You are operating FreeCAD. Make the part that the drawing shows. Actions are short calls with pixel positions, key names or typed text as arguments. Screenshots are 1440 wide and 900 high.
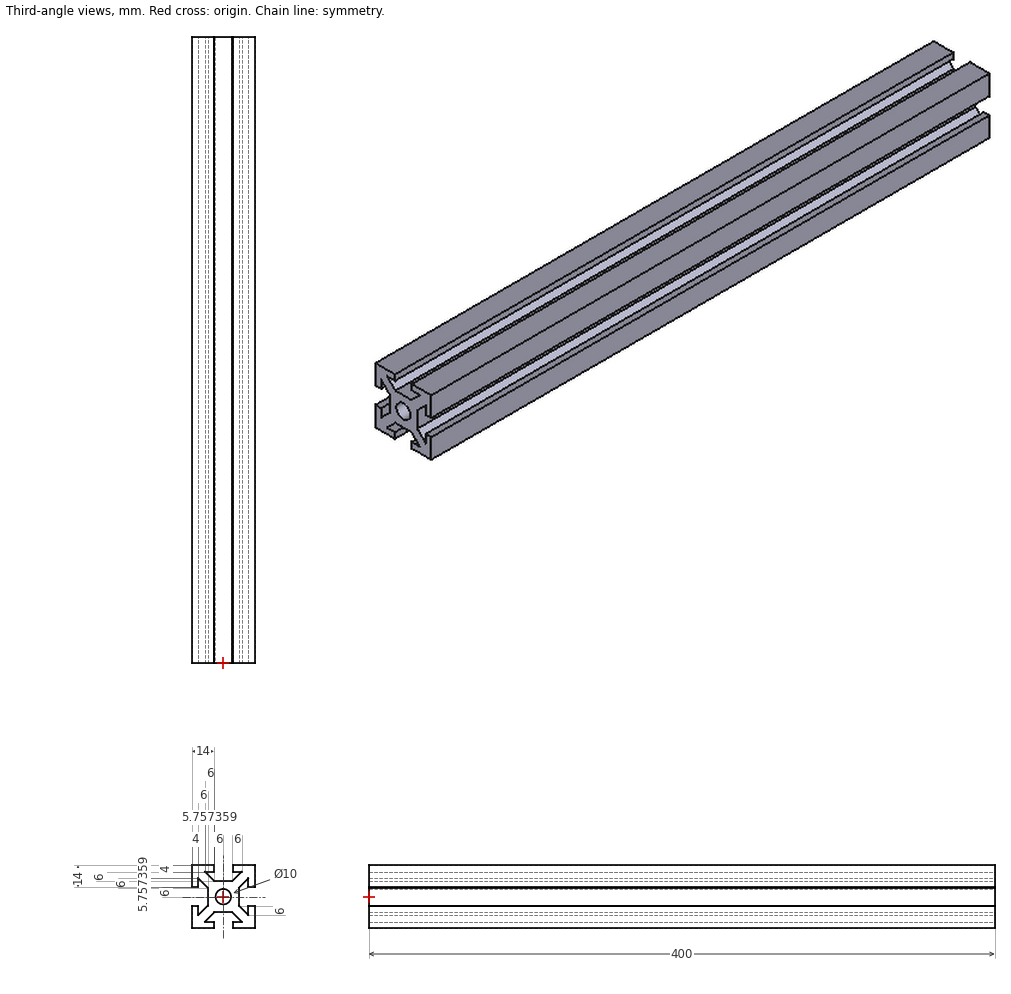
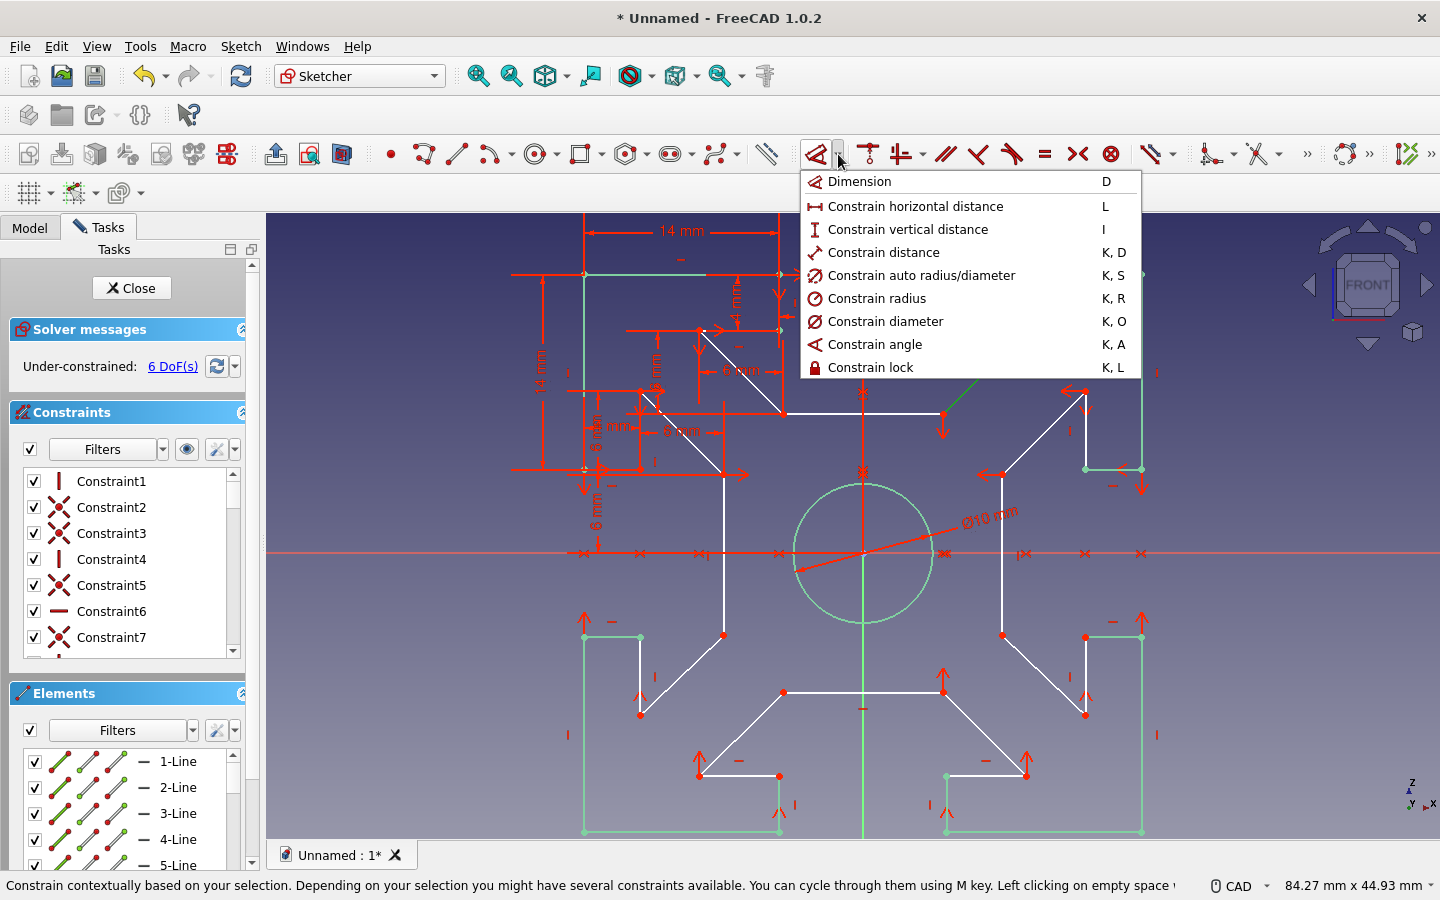
click(971, 206)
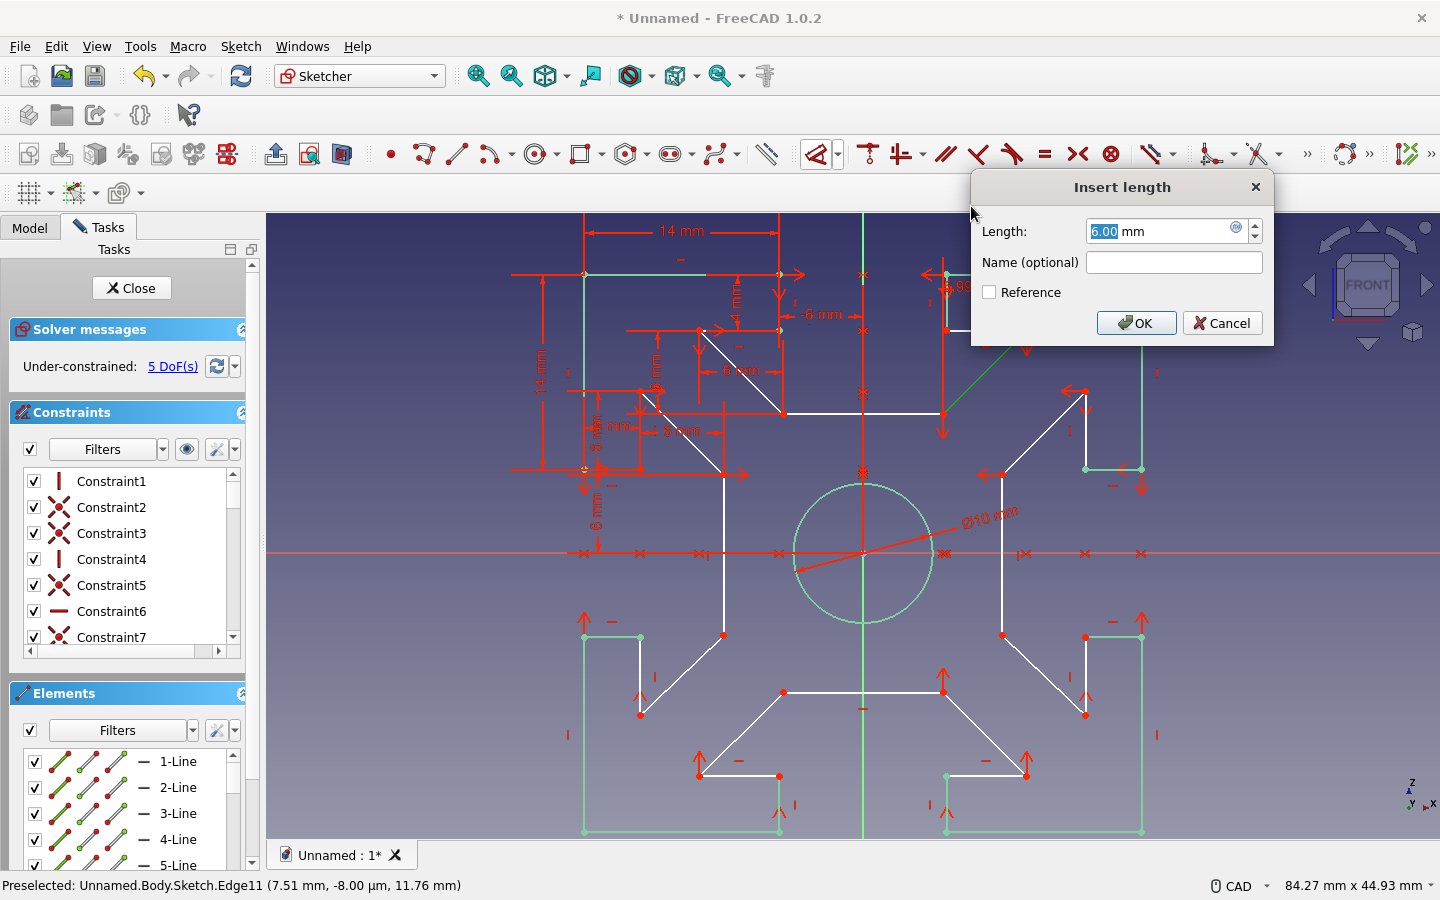
text(6)
key(Return)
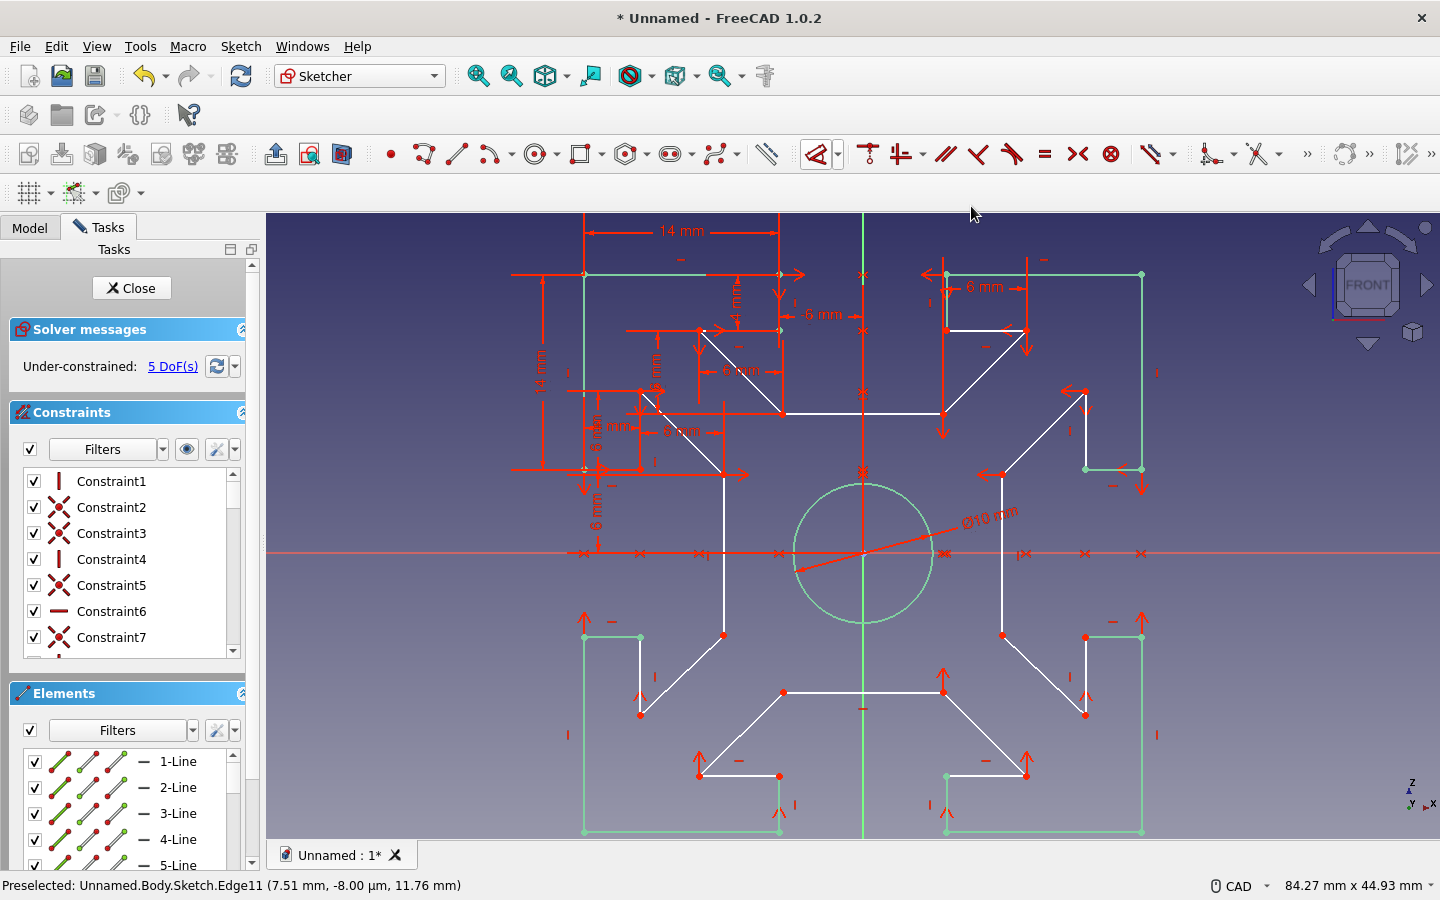
click(1027, 660)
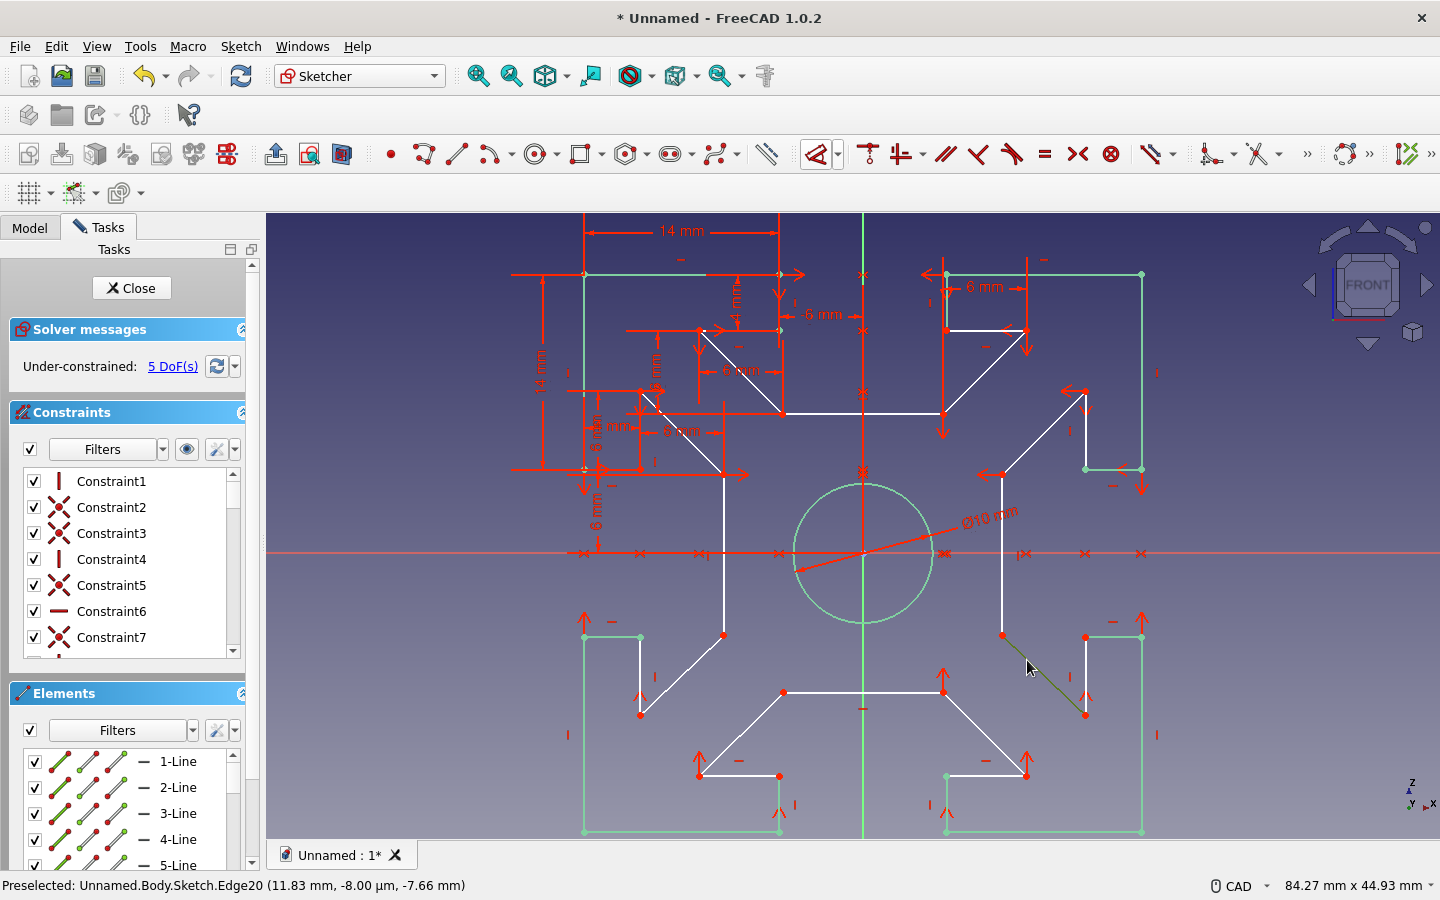
key(i)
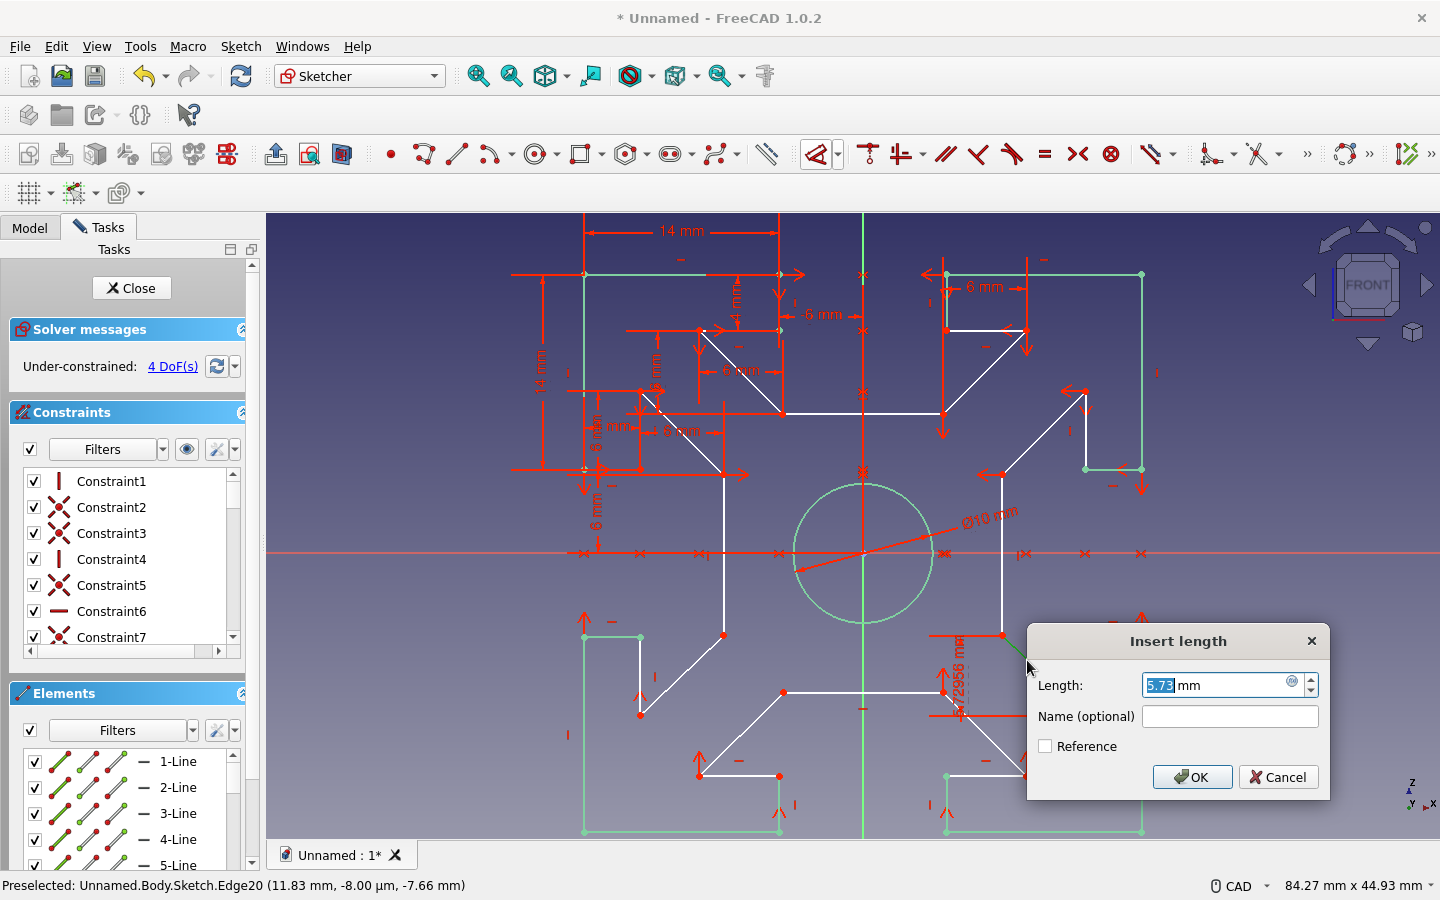
text(6)
key(Return)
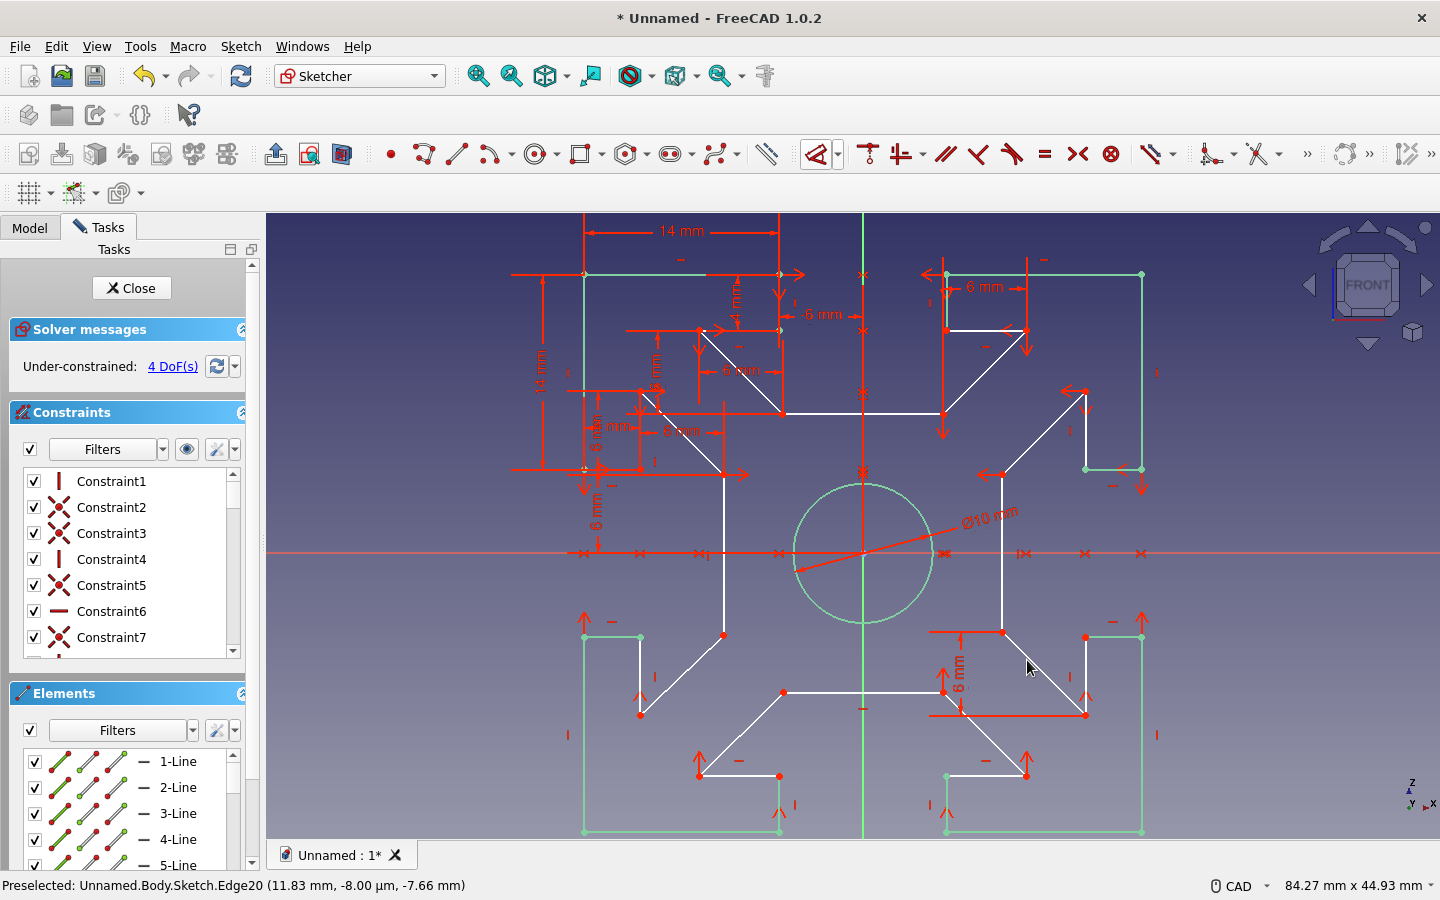
click(758, 718)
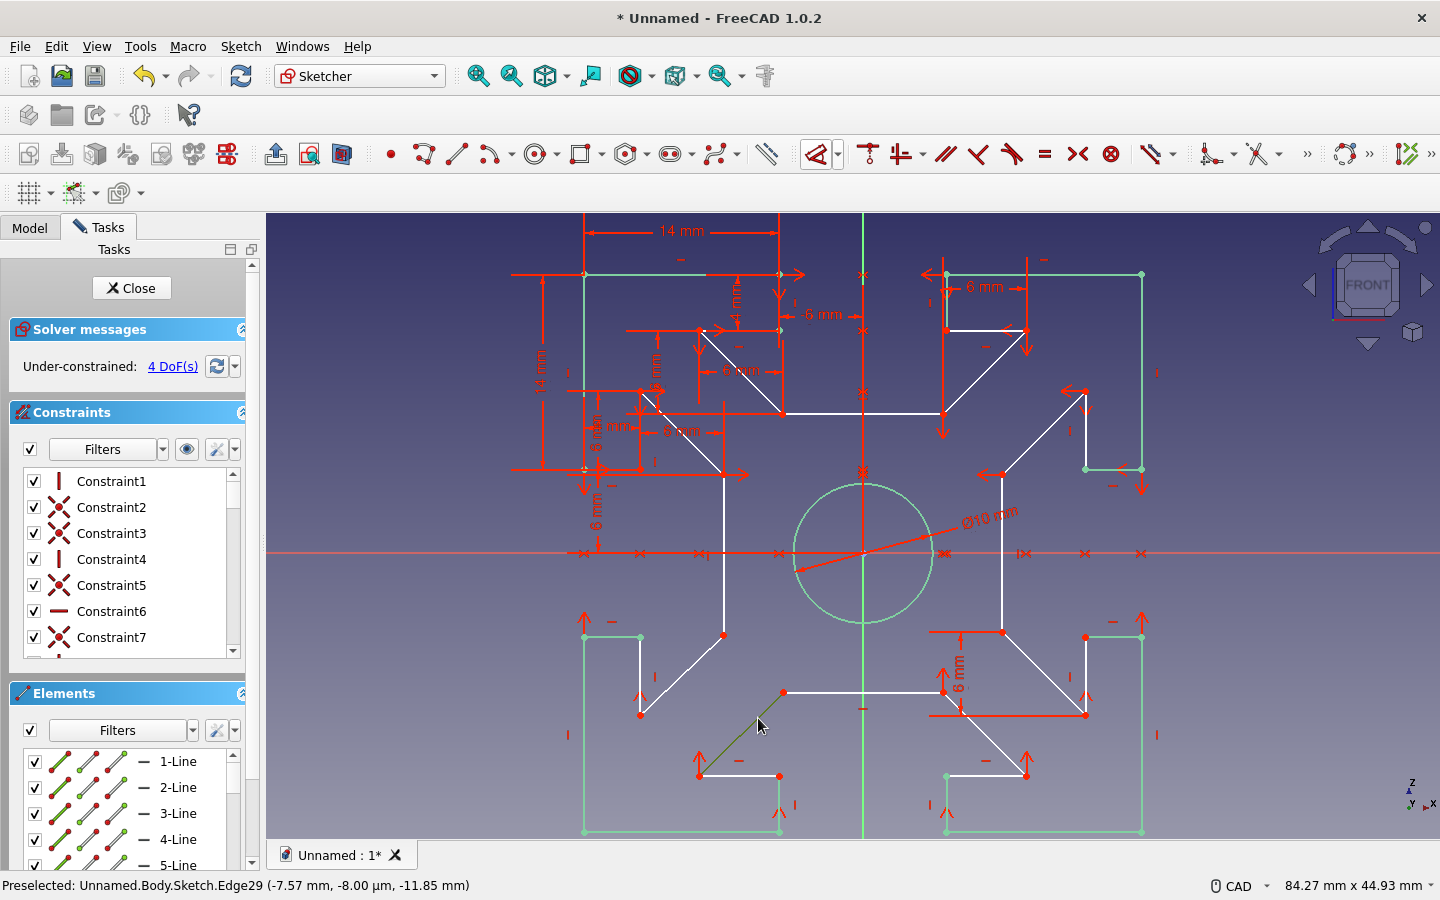
key(l)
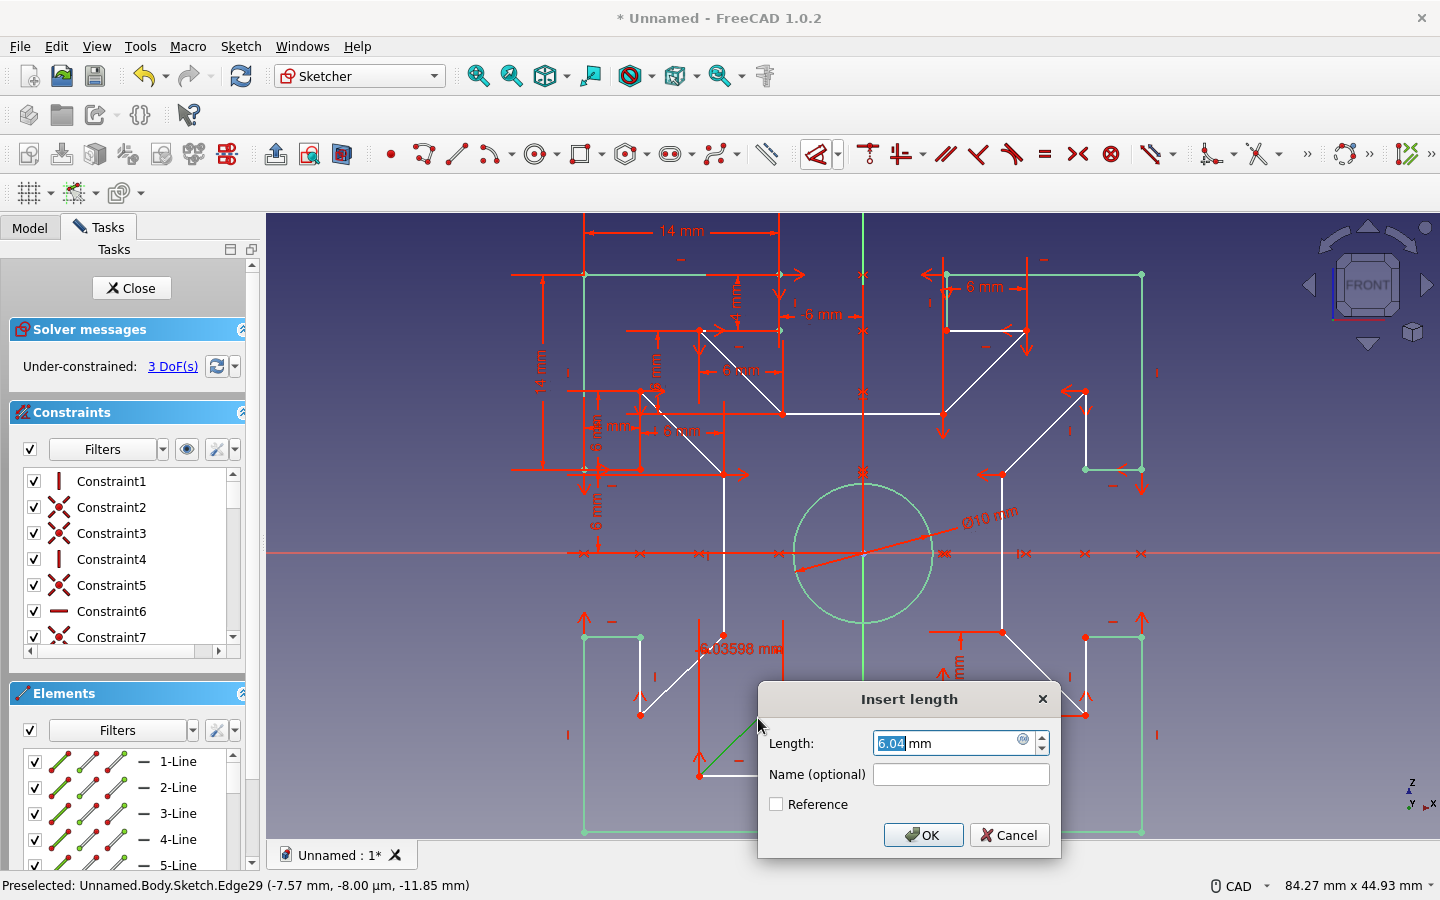
text(6)
key(Return)